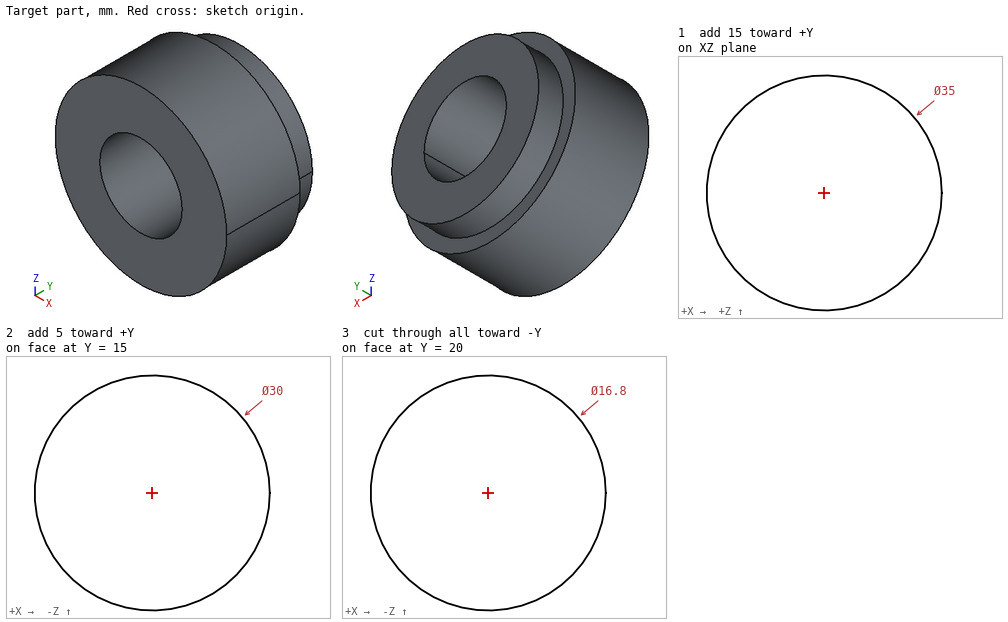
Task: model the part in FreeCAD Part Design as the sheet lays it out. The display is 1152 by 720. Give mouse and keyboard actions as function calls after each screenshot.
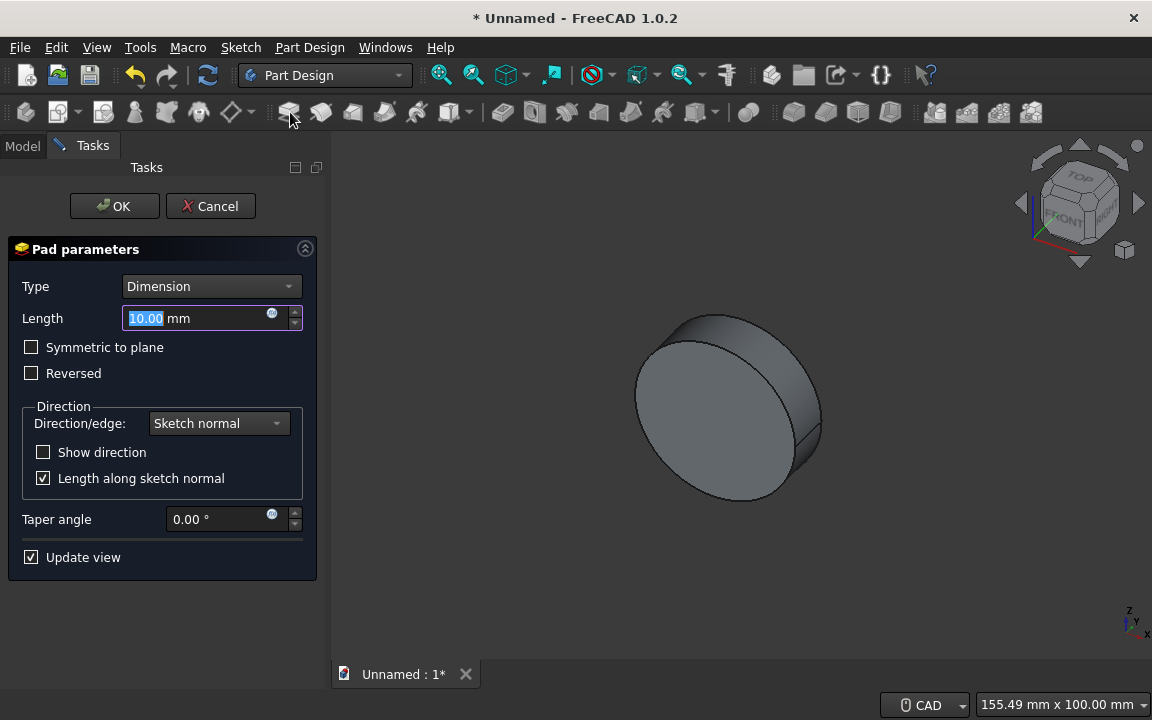
text(15)
key(Tab)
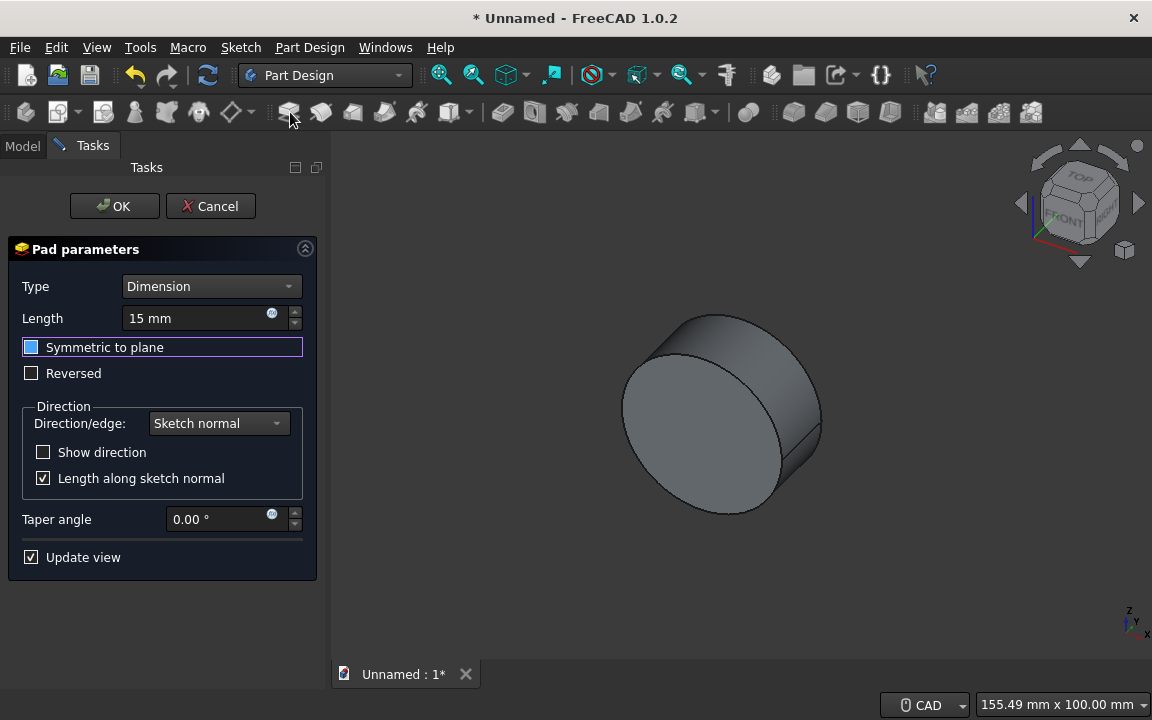
click(30, 373)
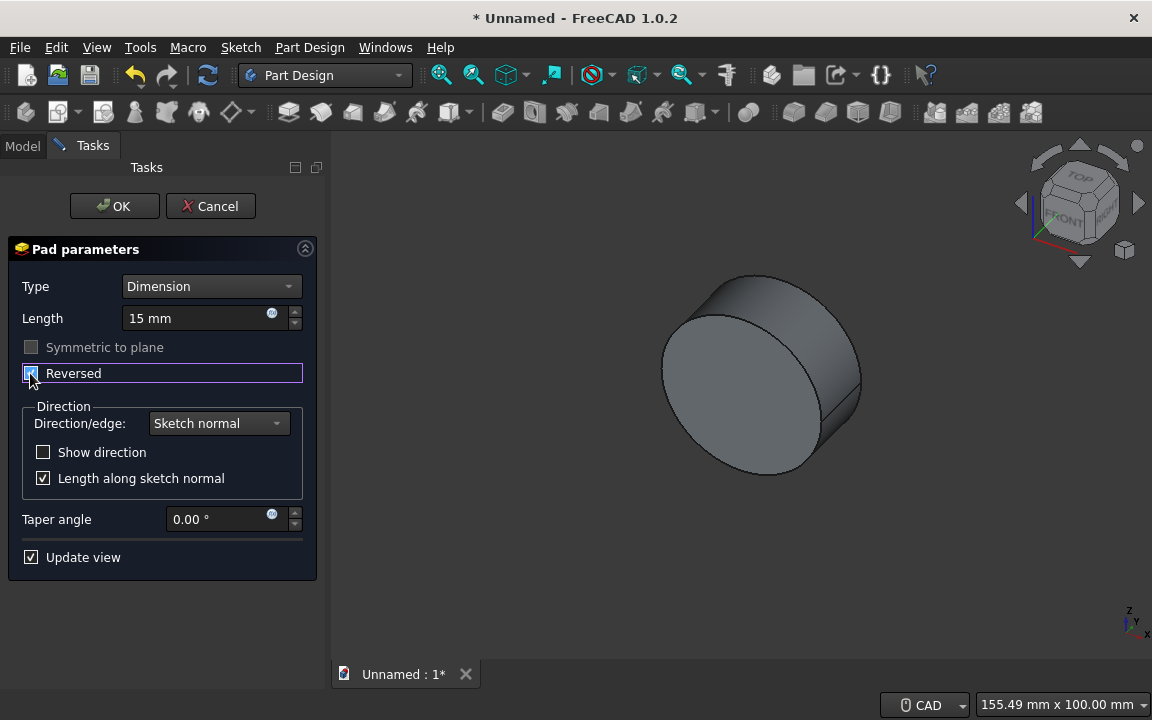
click(115, 206)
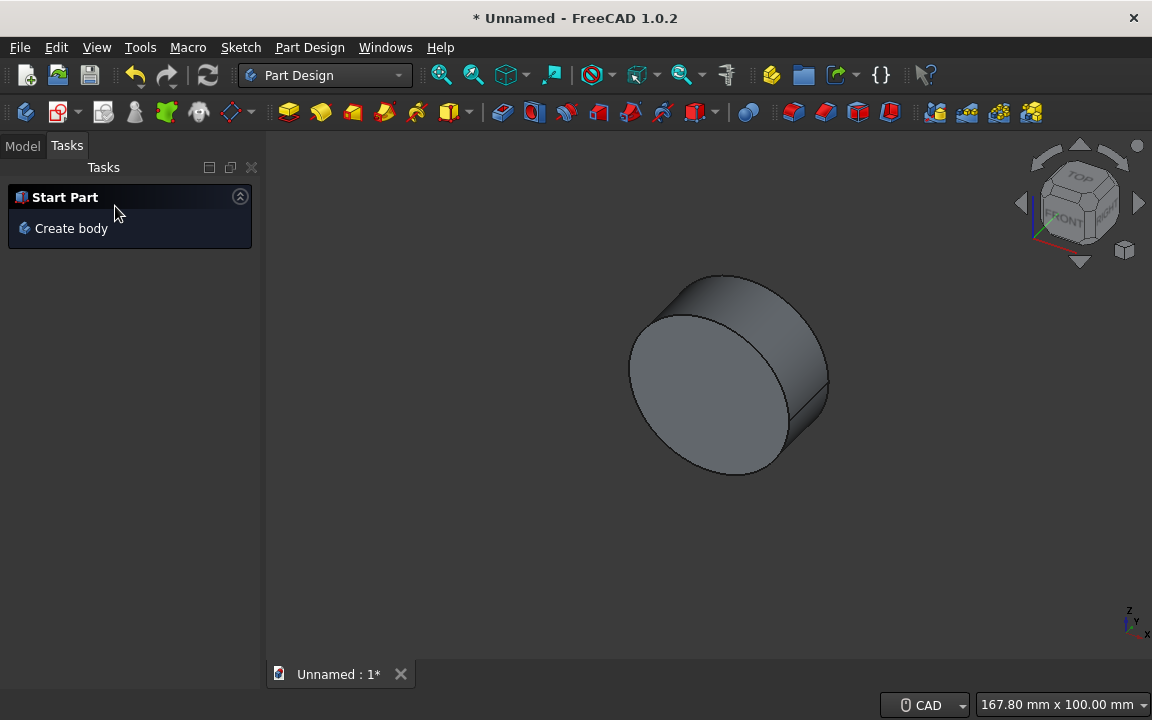
key(4)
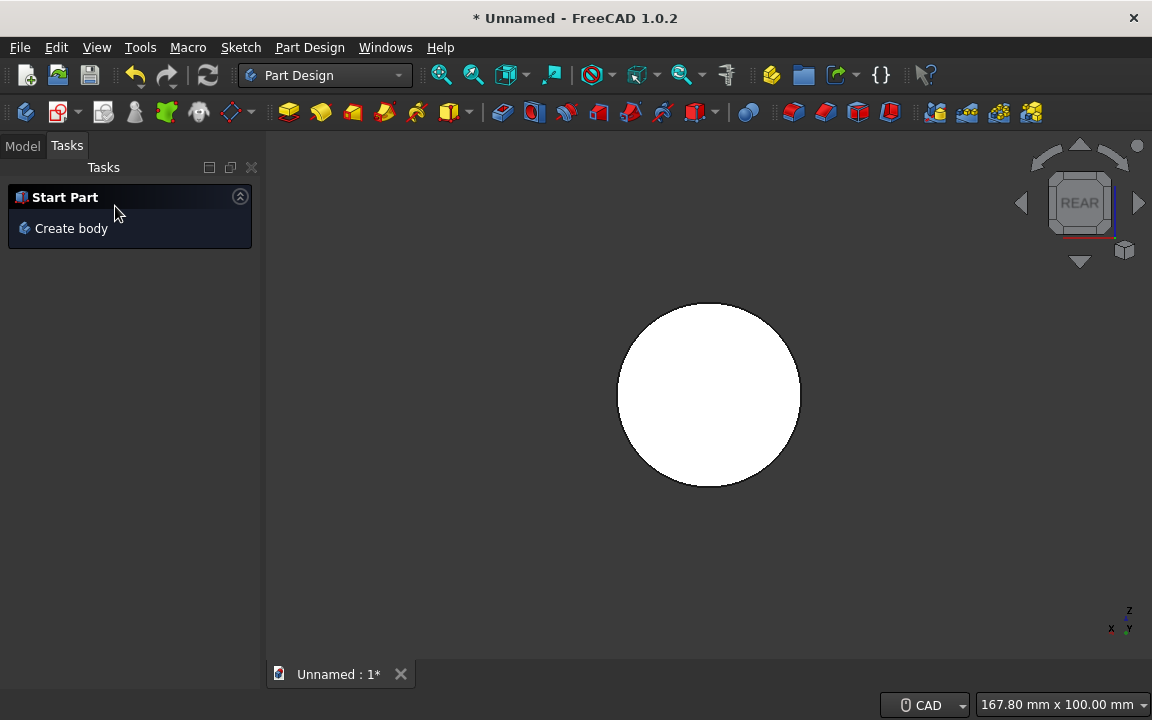
click(442, 76)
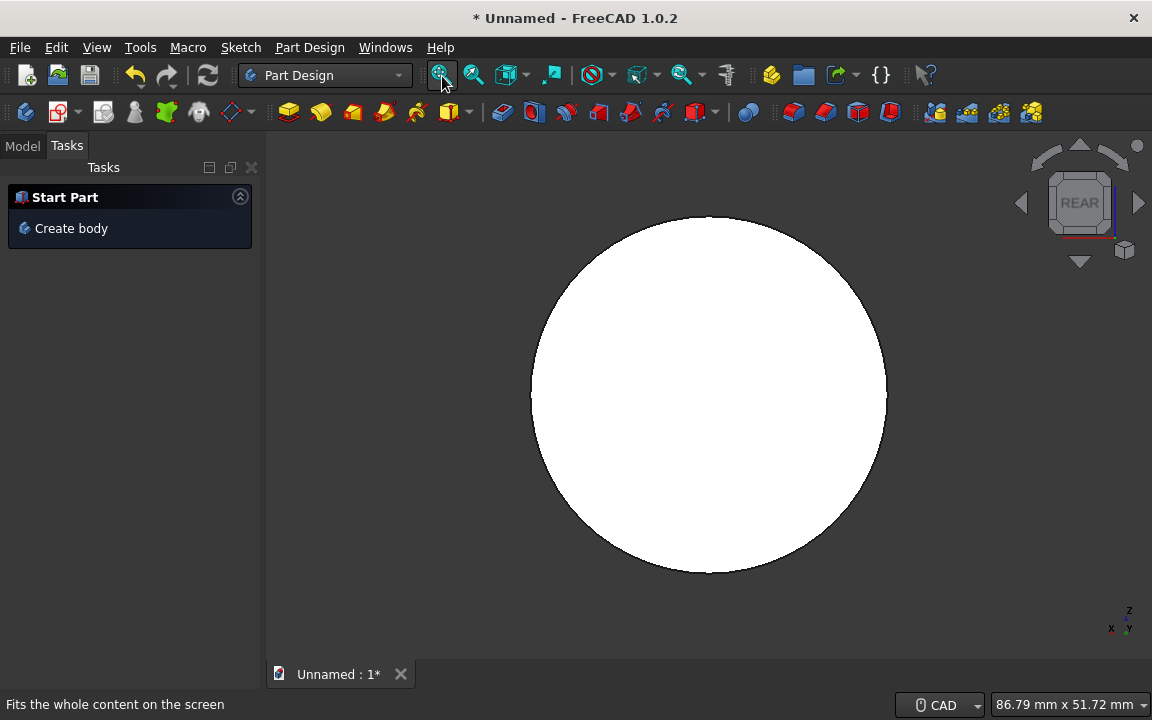
click(709, 394)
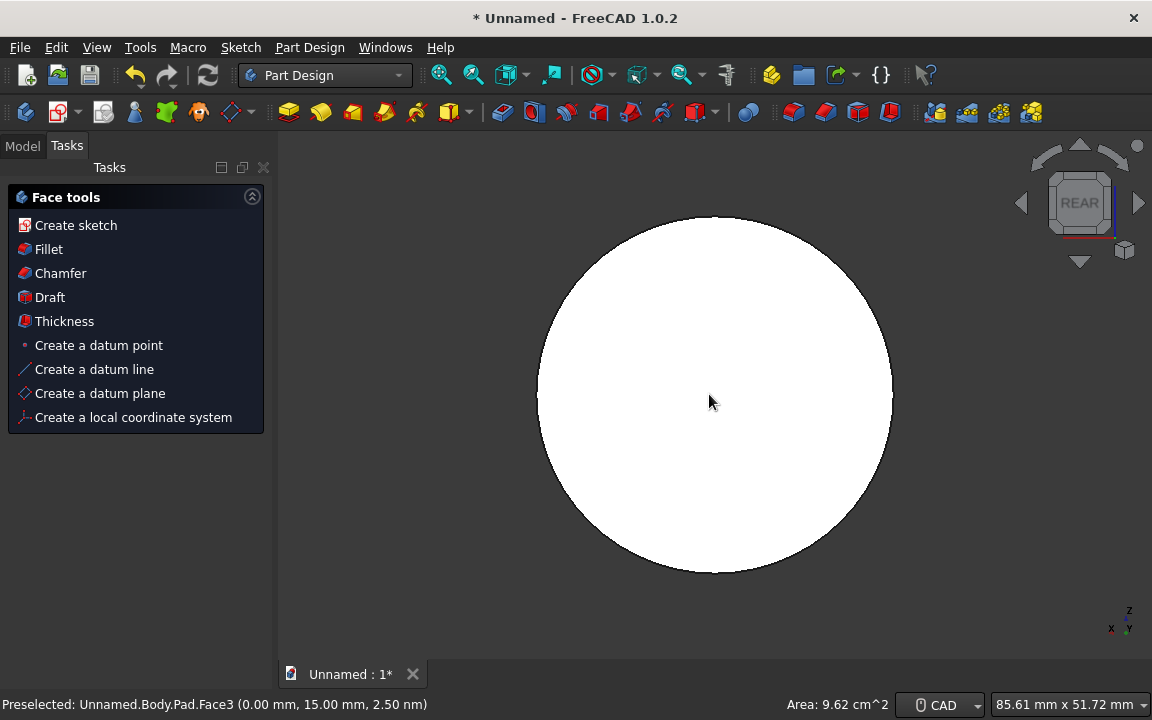
click(58, 112)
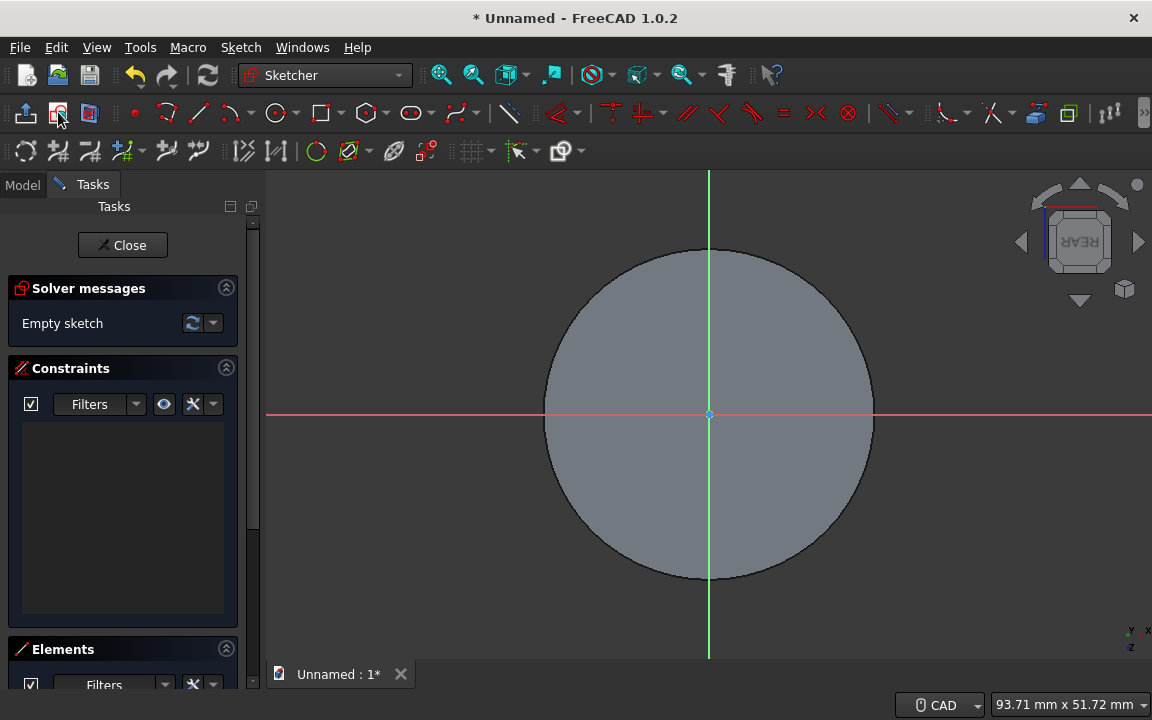
click(276, 114)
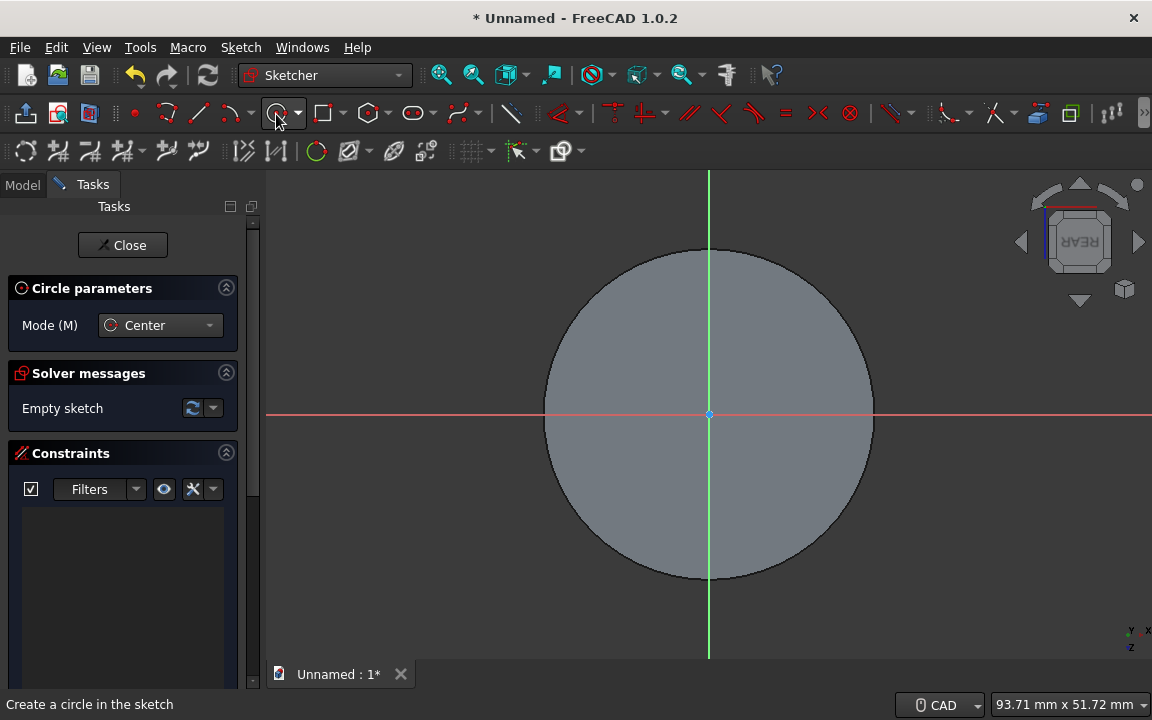
click(709, 414)
click(809, 314)
key(Escape)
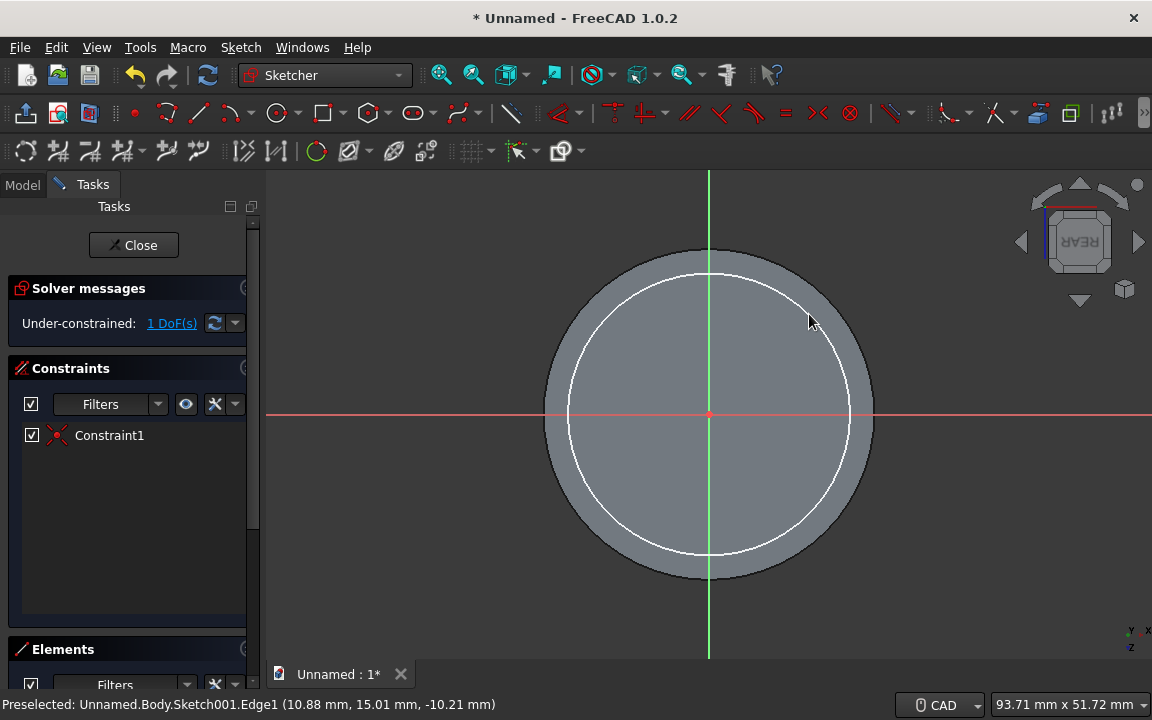
click(558, 114)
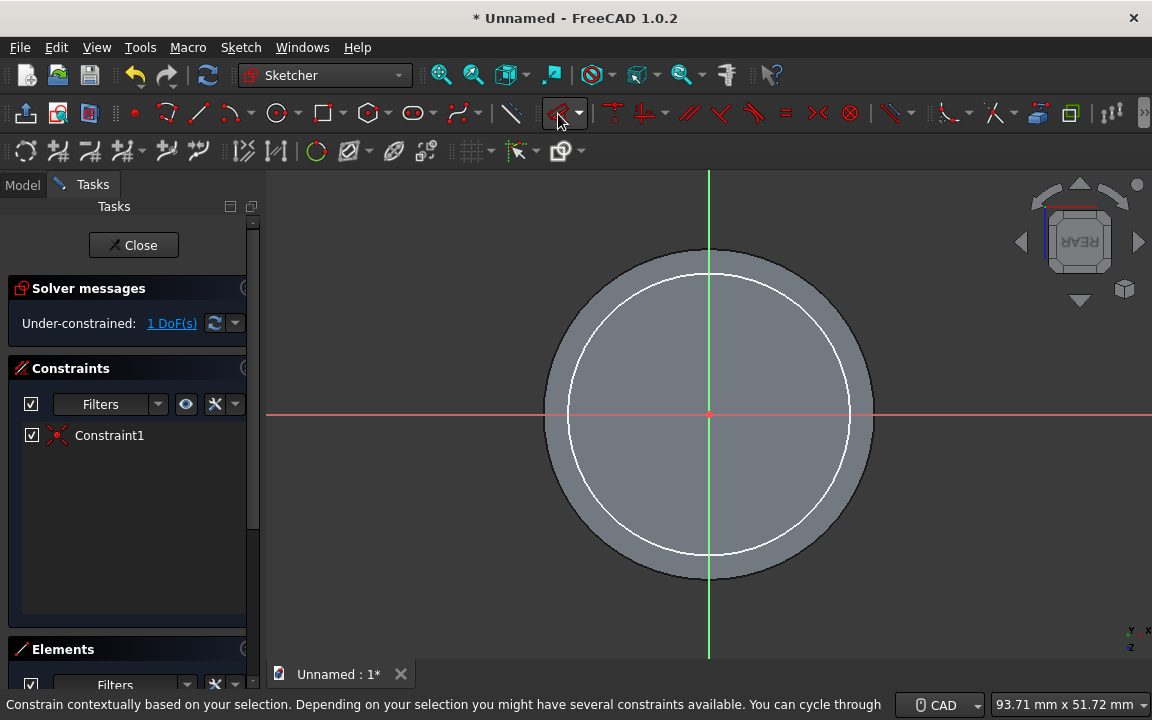
click(808, 314)
click(830, 291)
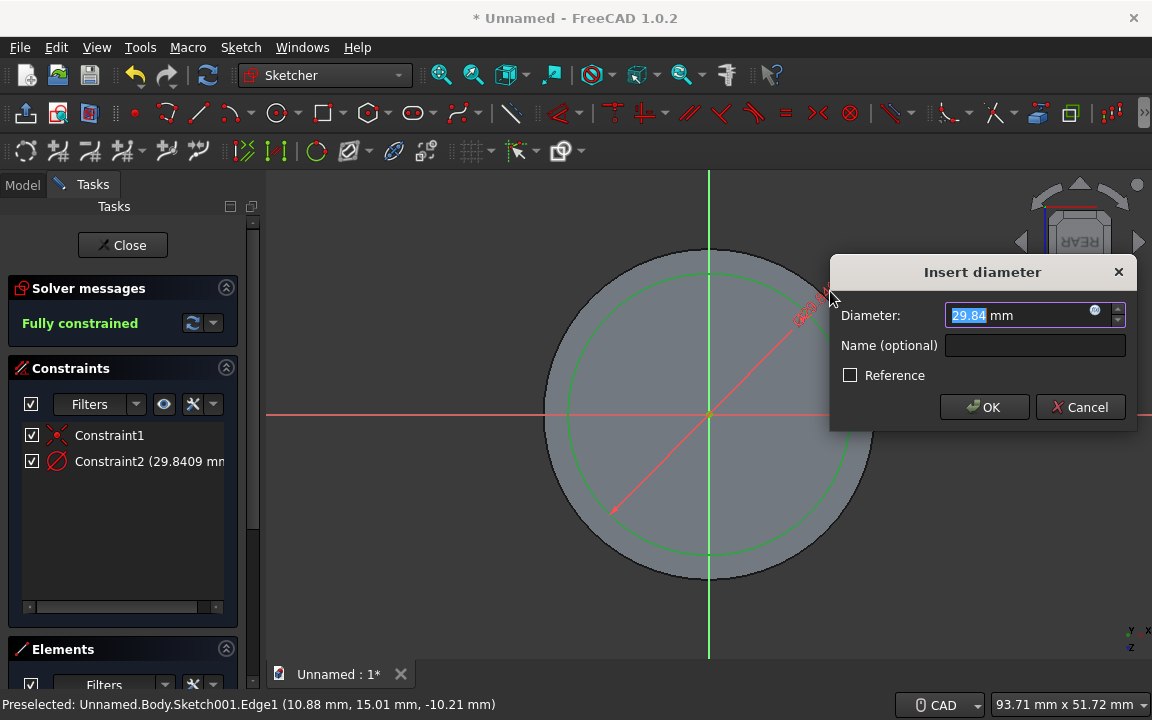
text(30)
key(Return)
key(Escape)